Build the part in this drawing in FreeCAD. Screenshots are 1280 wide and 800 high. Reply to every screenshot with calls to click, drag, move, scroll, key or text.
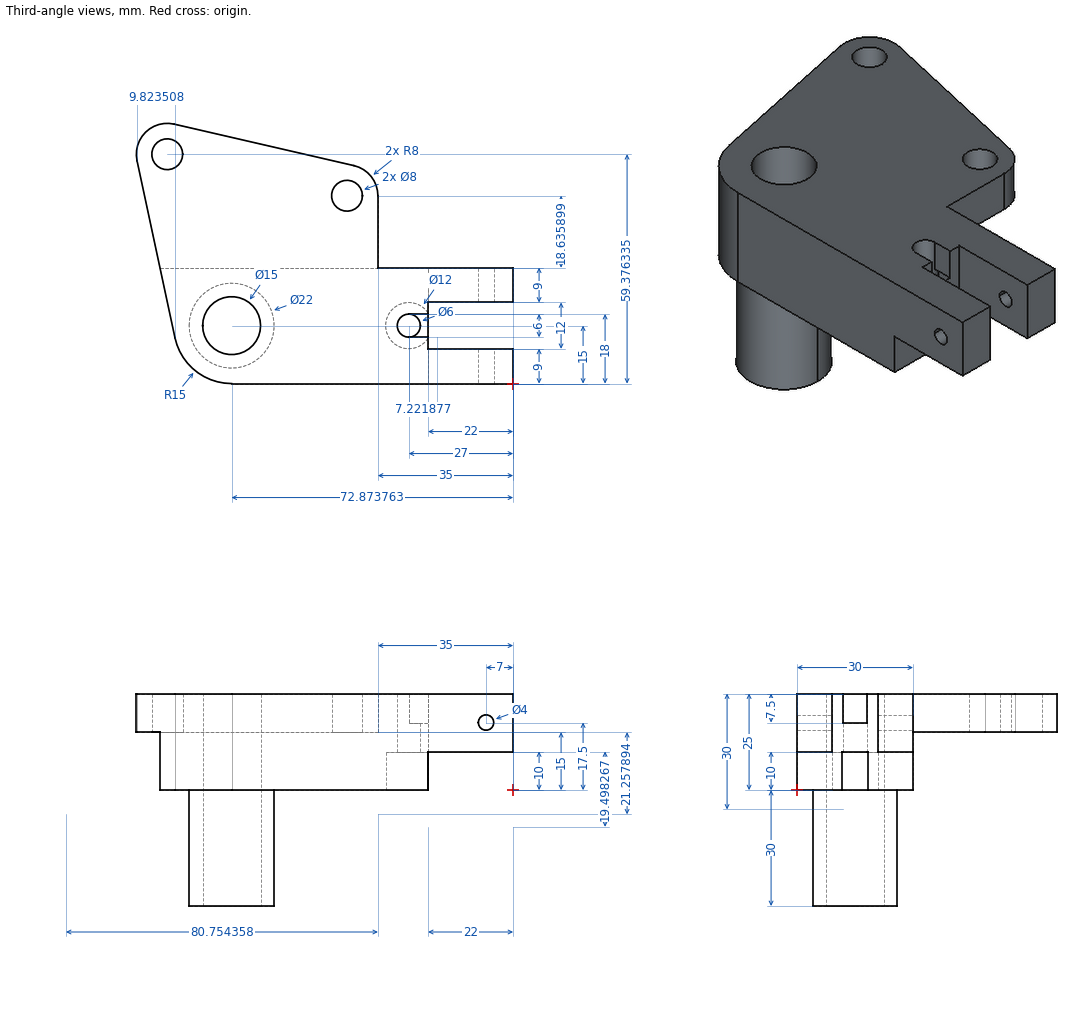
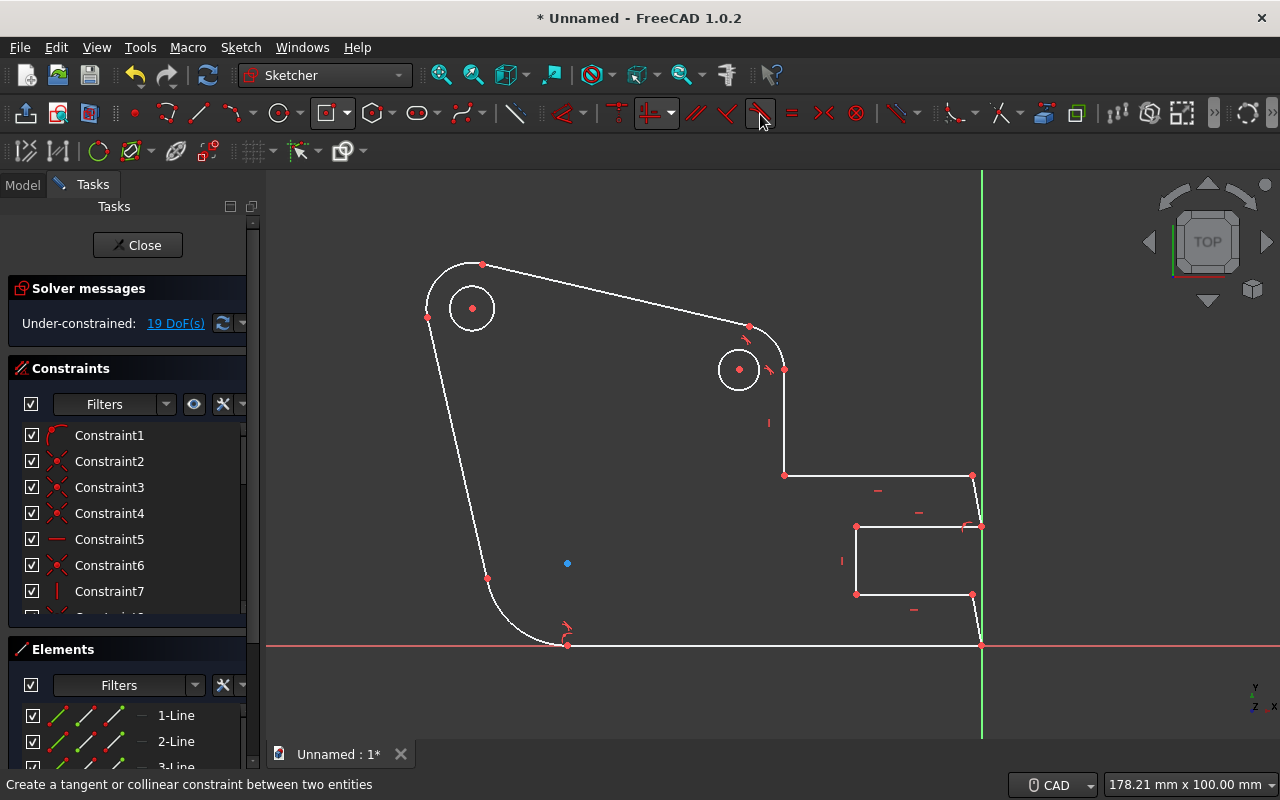
click(669, 307)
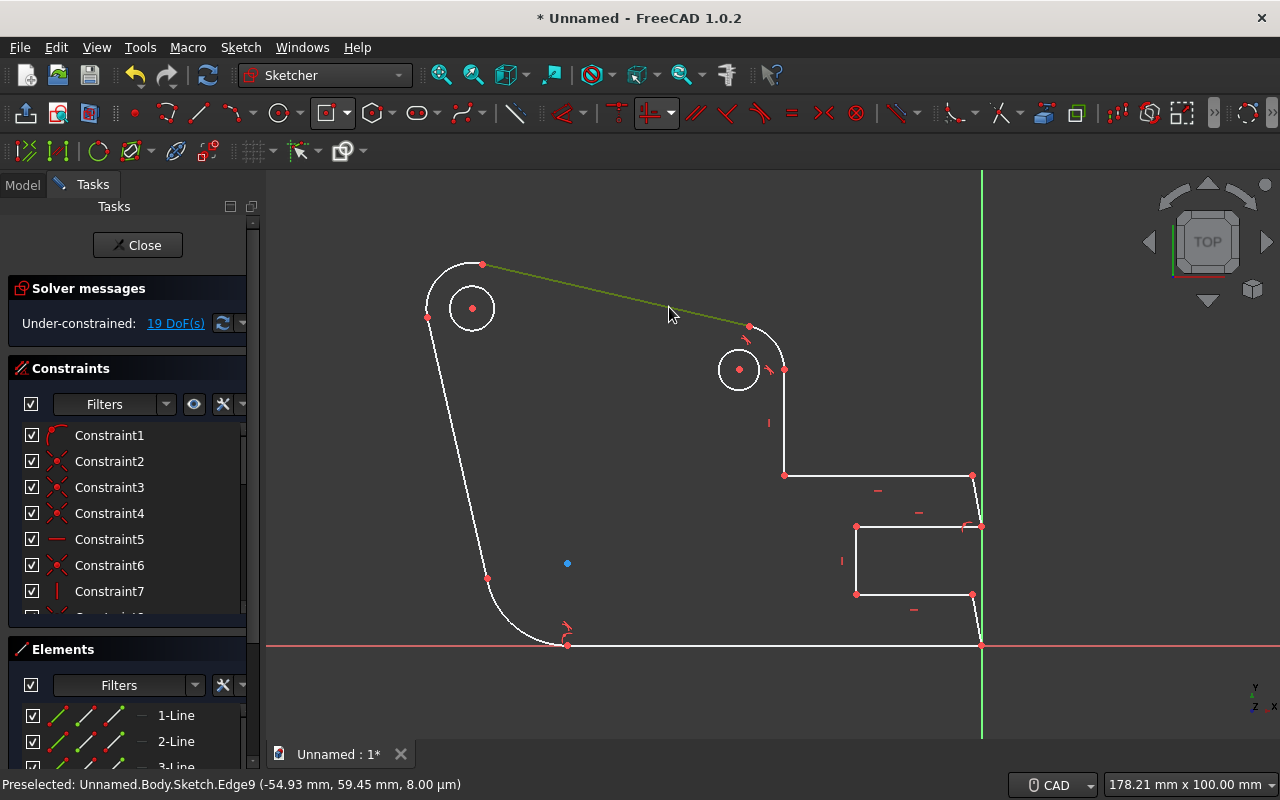
click(455, 266)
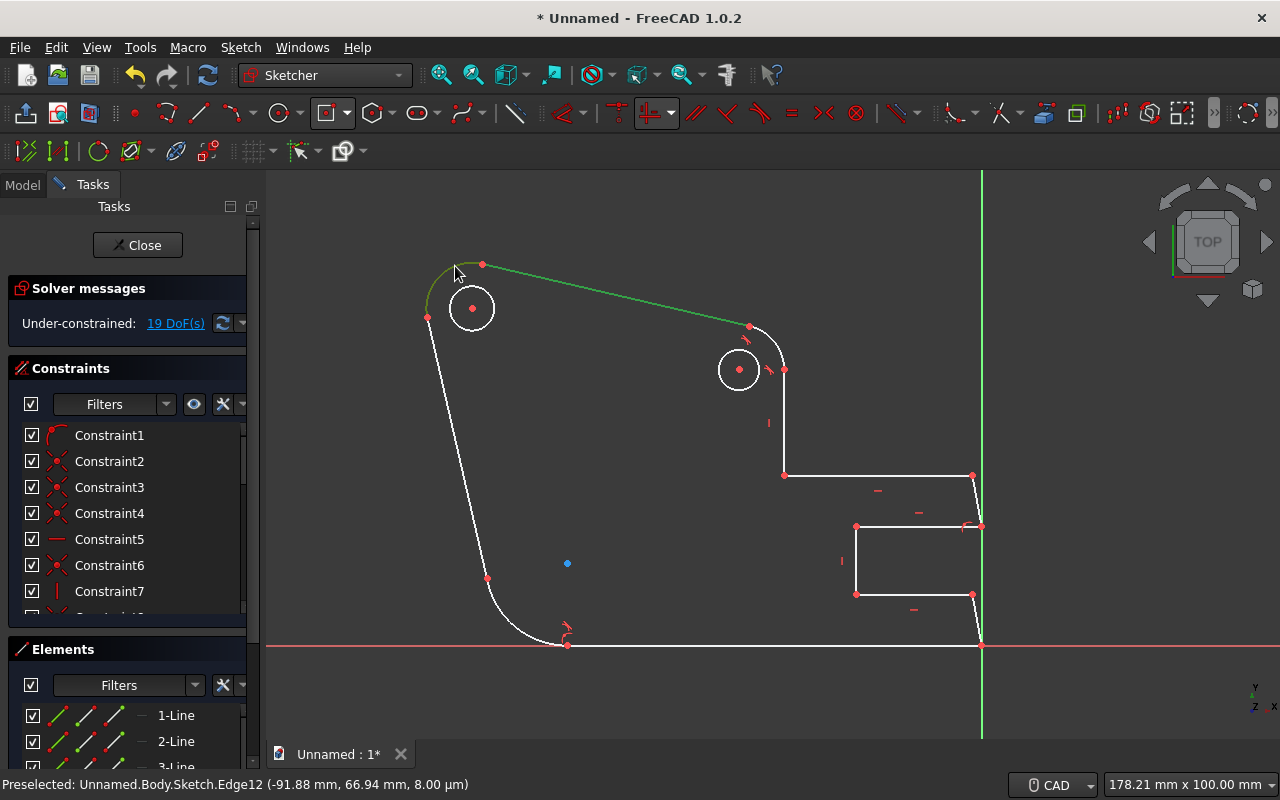
click(760, 114)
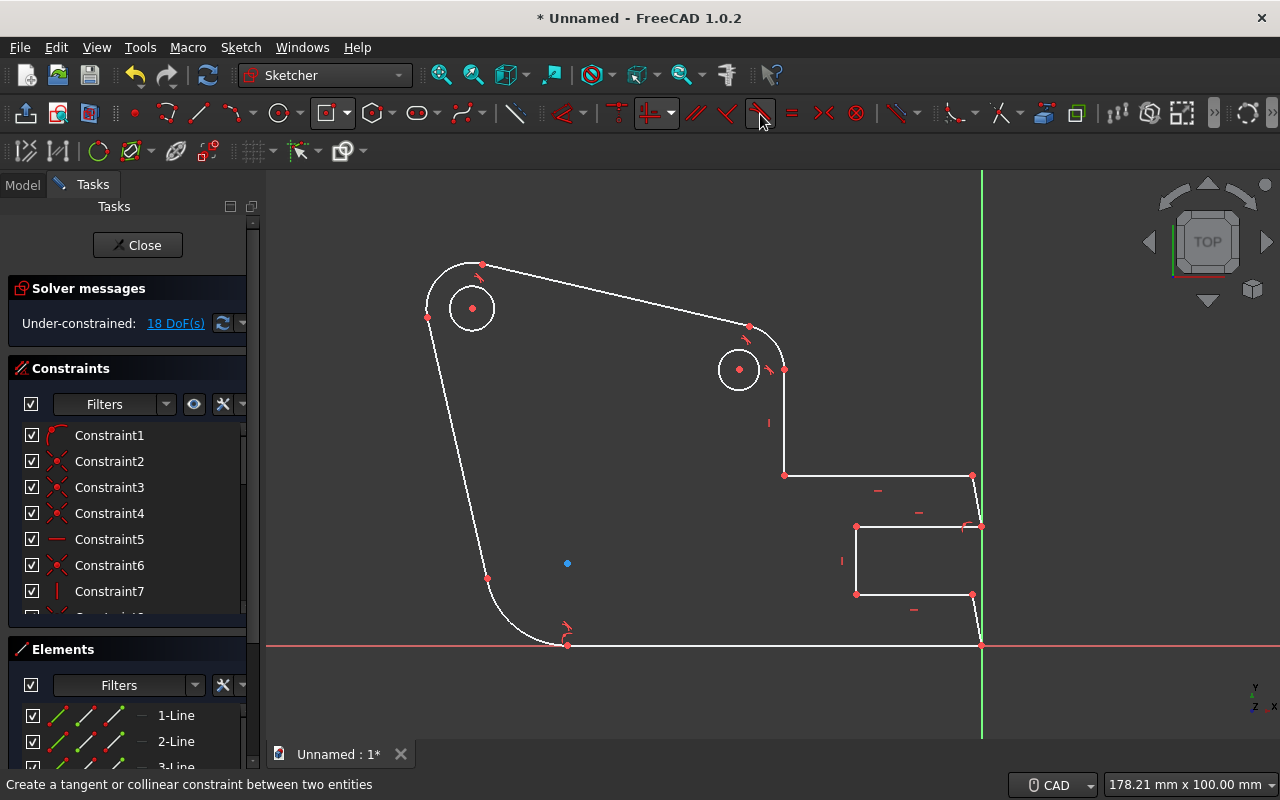
click(445, 396)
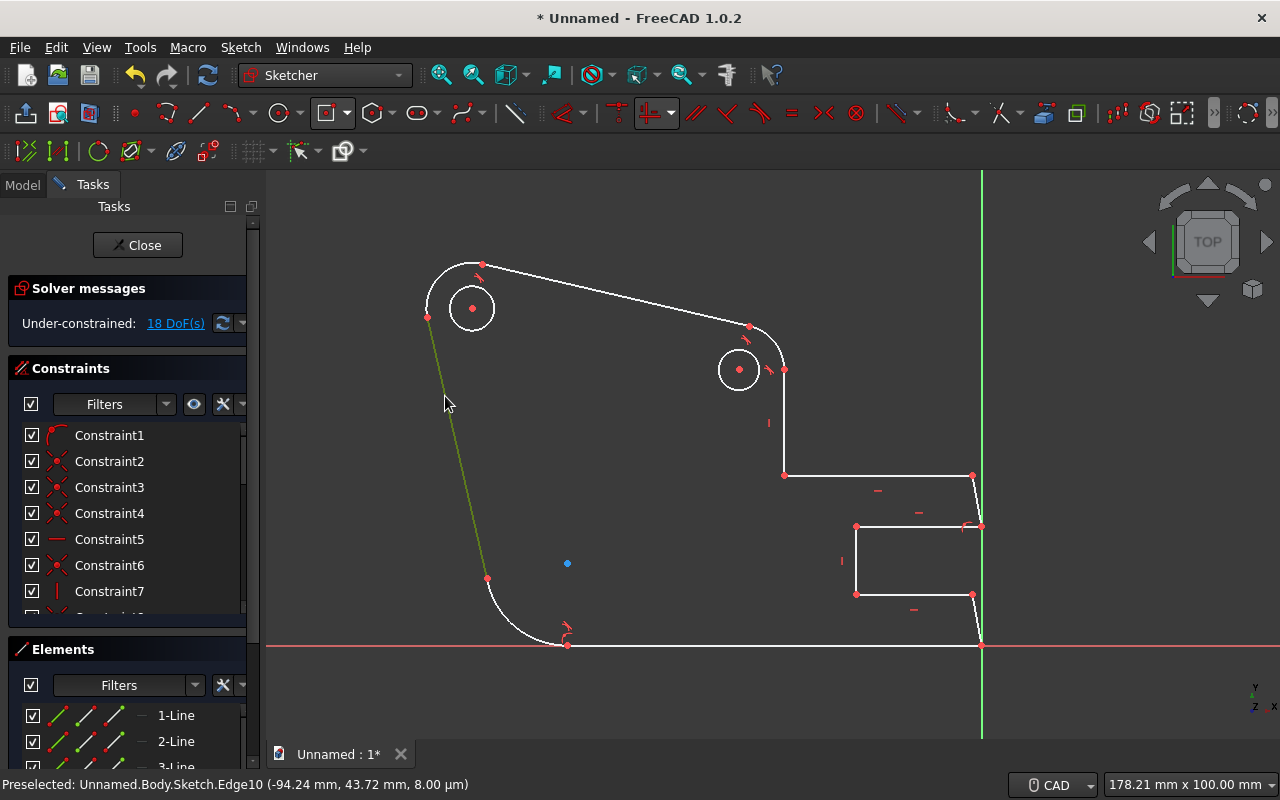
click(455, 266)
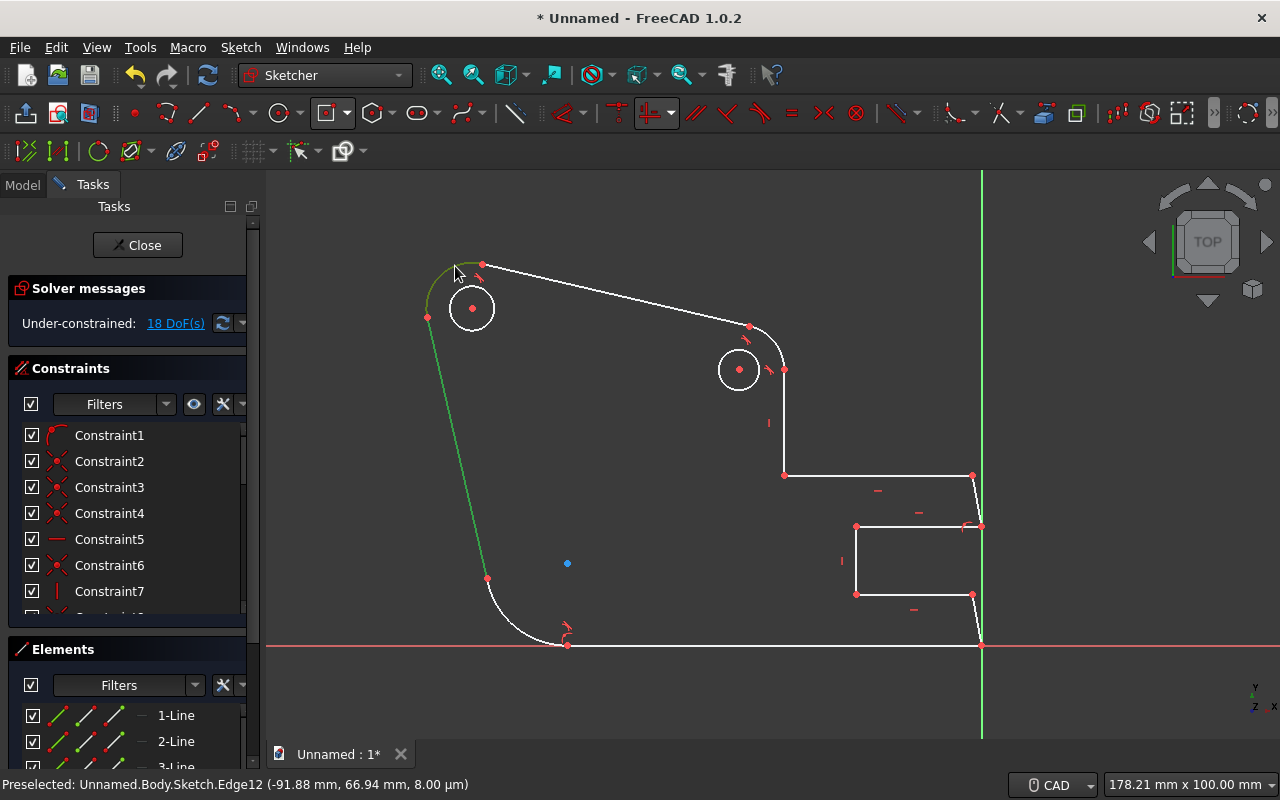
click(760, 114)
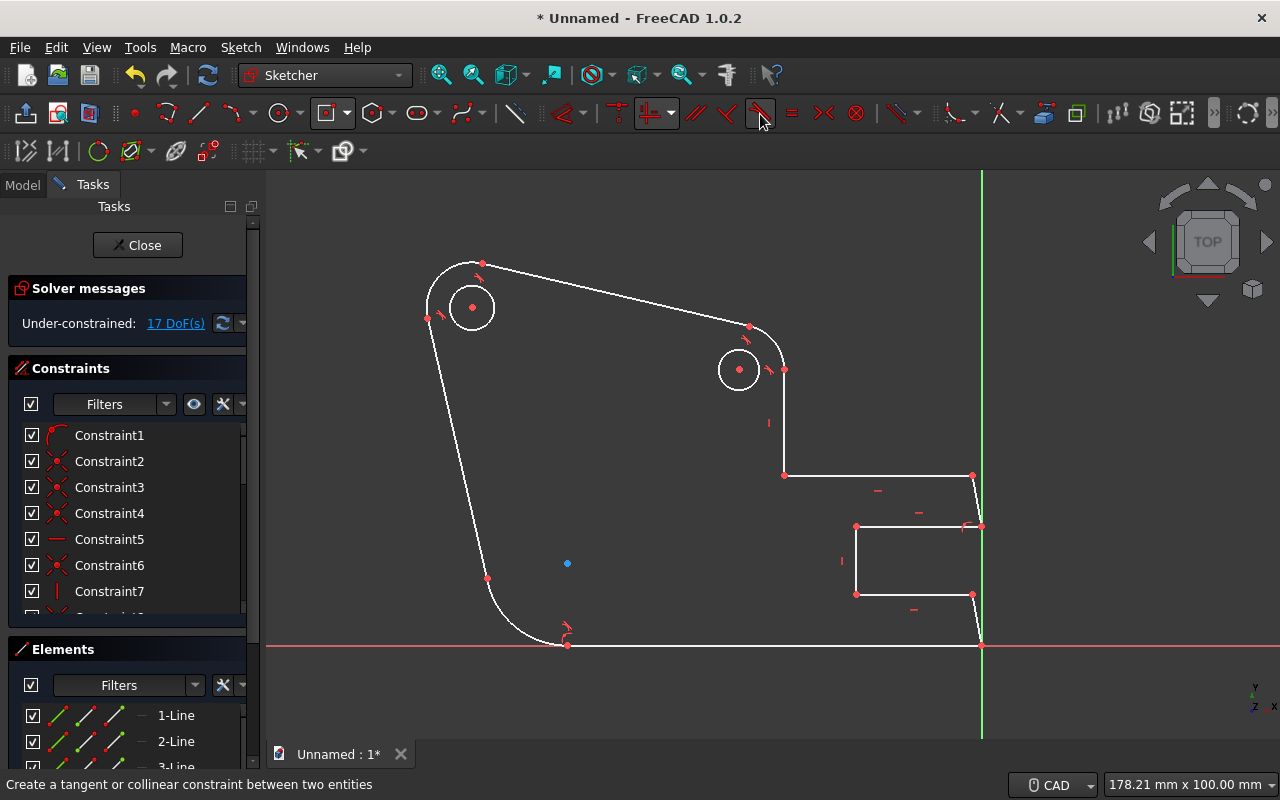
click(446, 396)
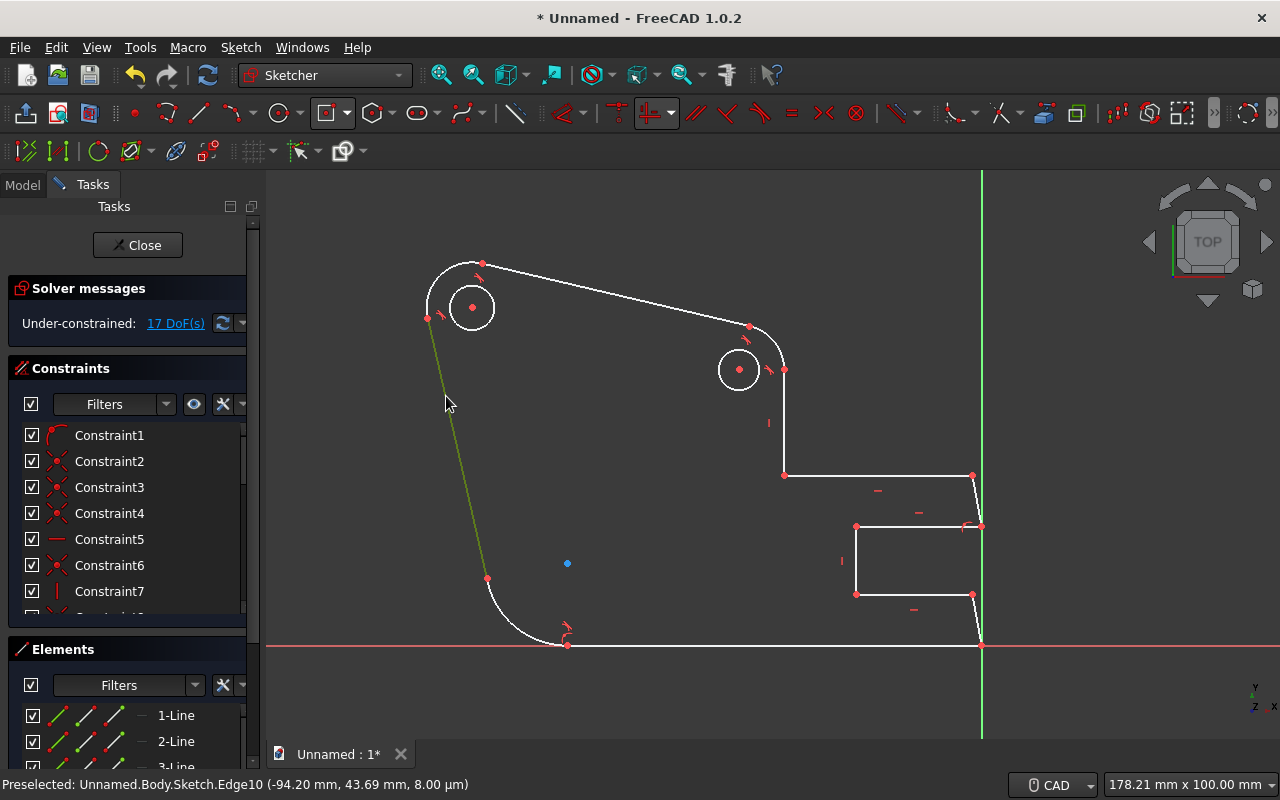
click(500, 610)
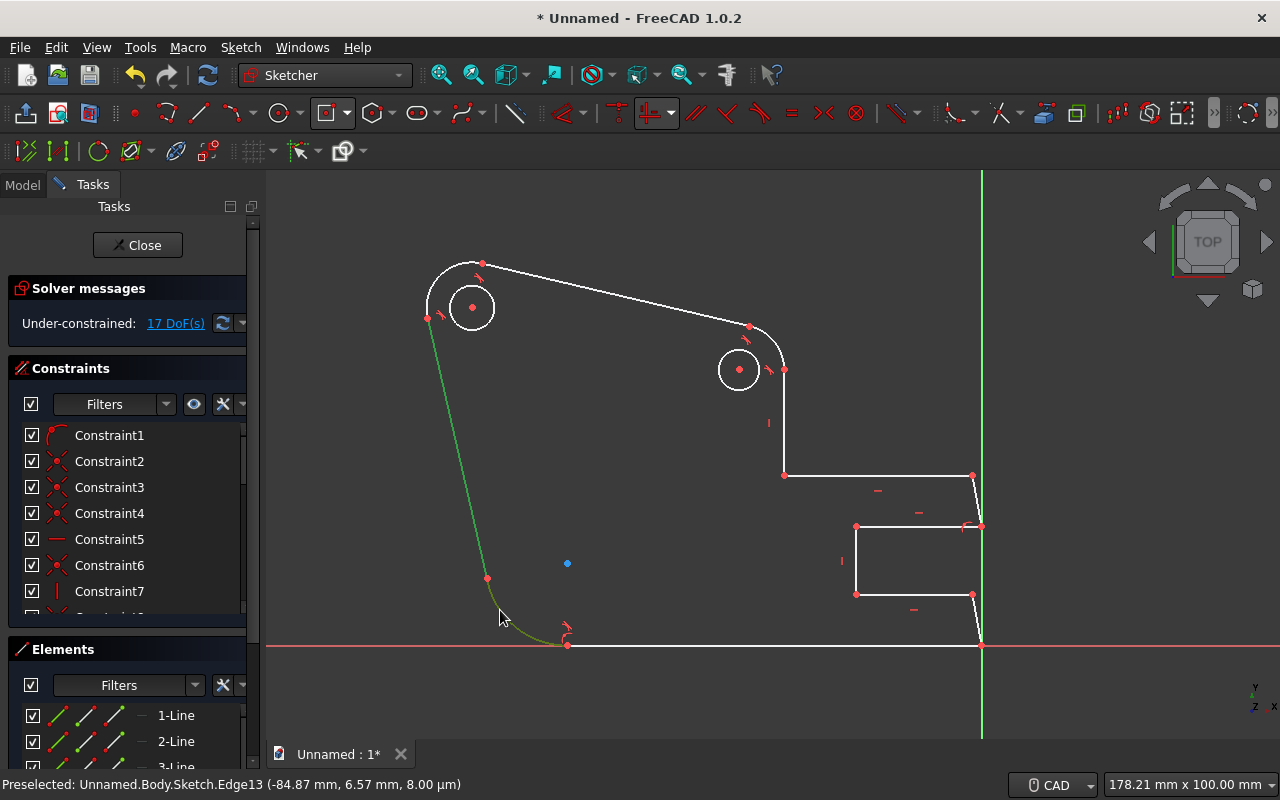
click(760, 114)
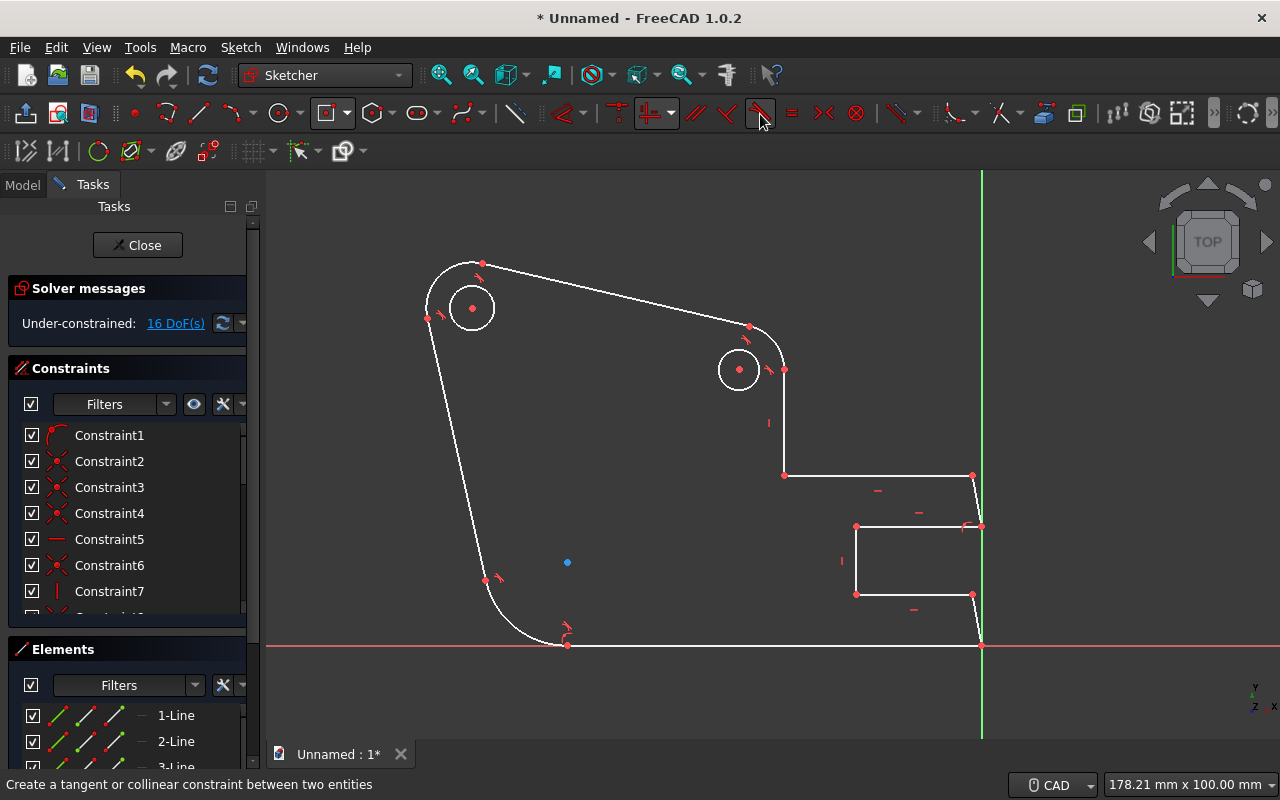
click(979, 630)